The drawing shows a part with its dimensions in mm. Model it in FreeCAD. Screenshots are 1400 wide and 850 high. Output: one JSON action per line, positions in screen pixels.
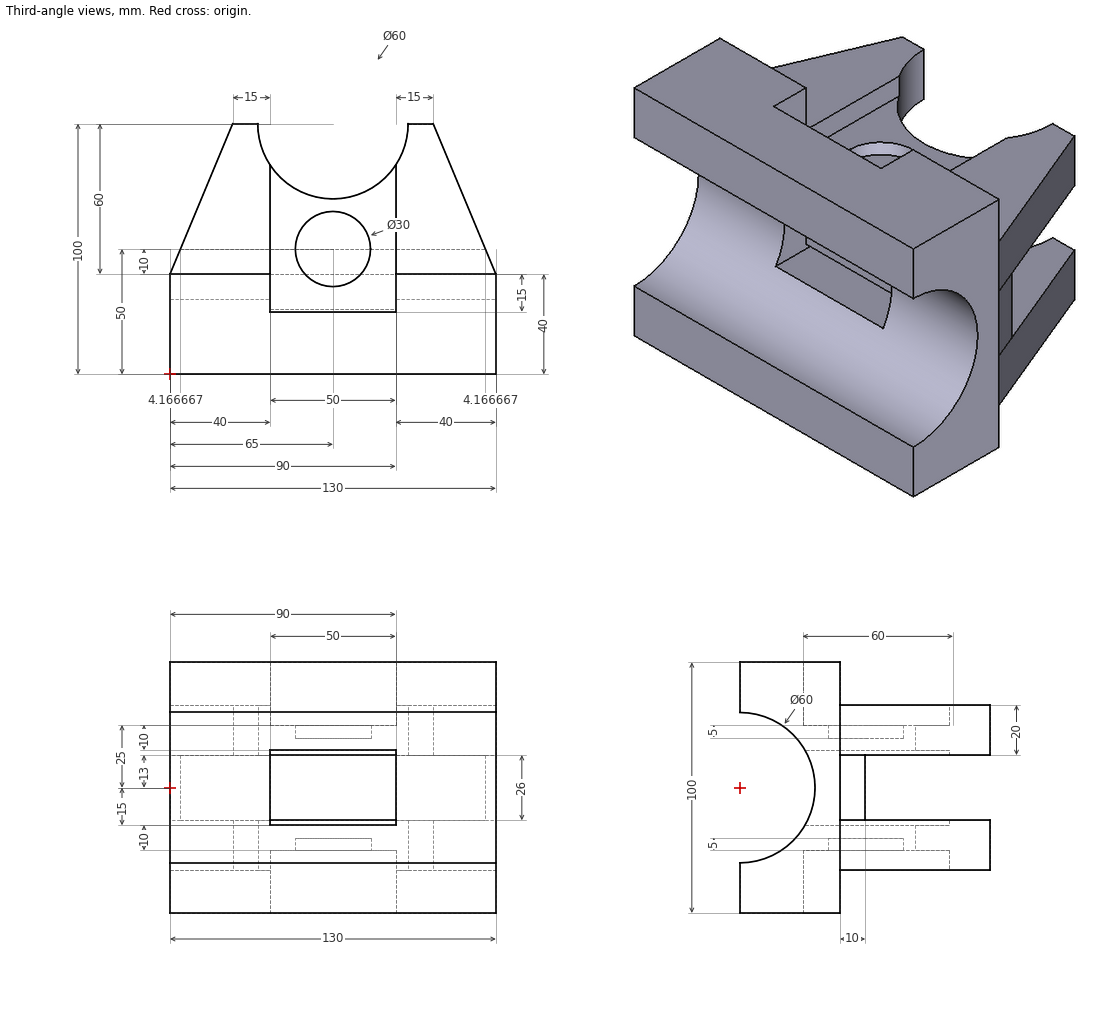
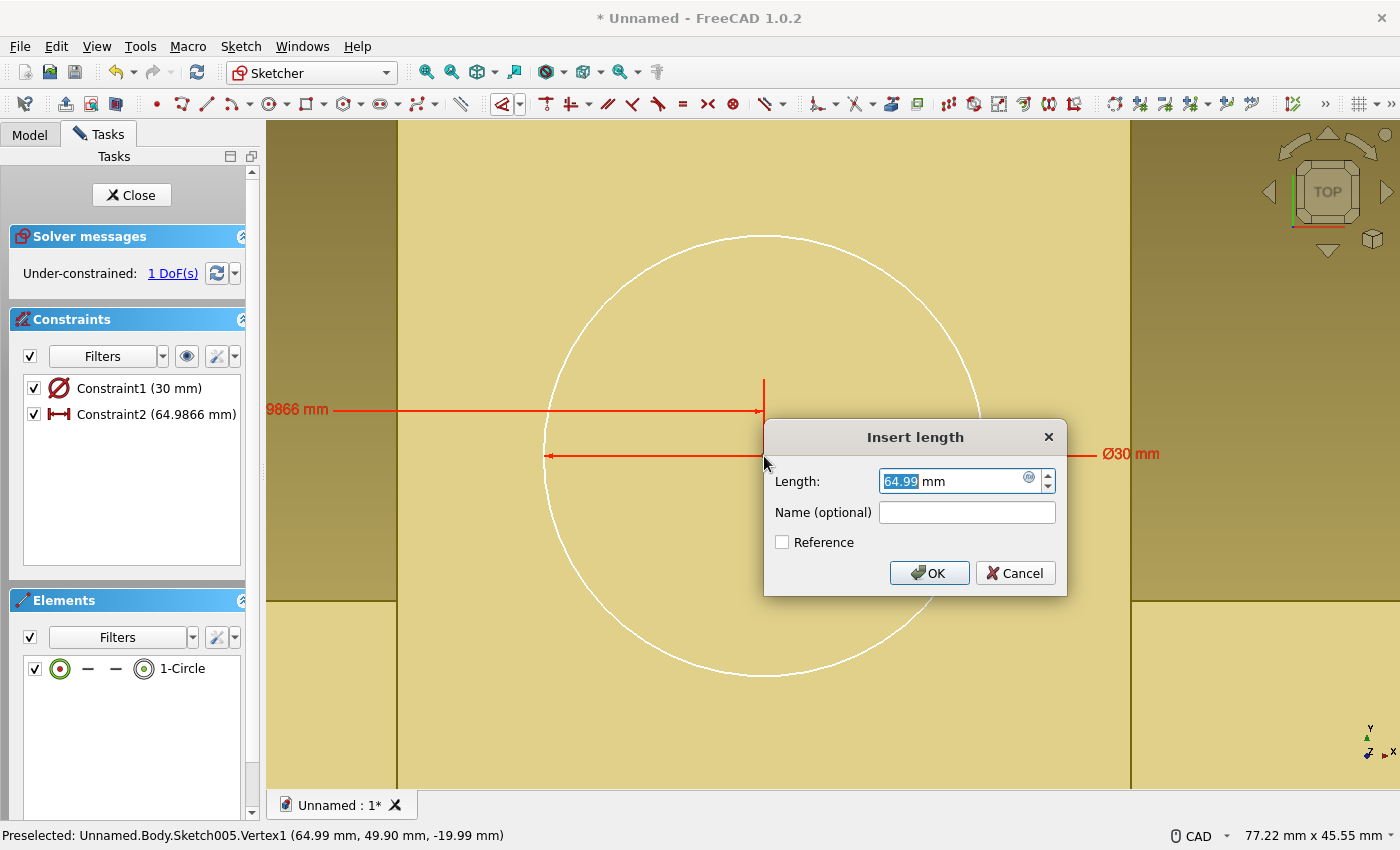
{"action": "type", "text": "65"}
{"action": "key", "text": "Return"}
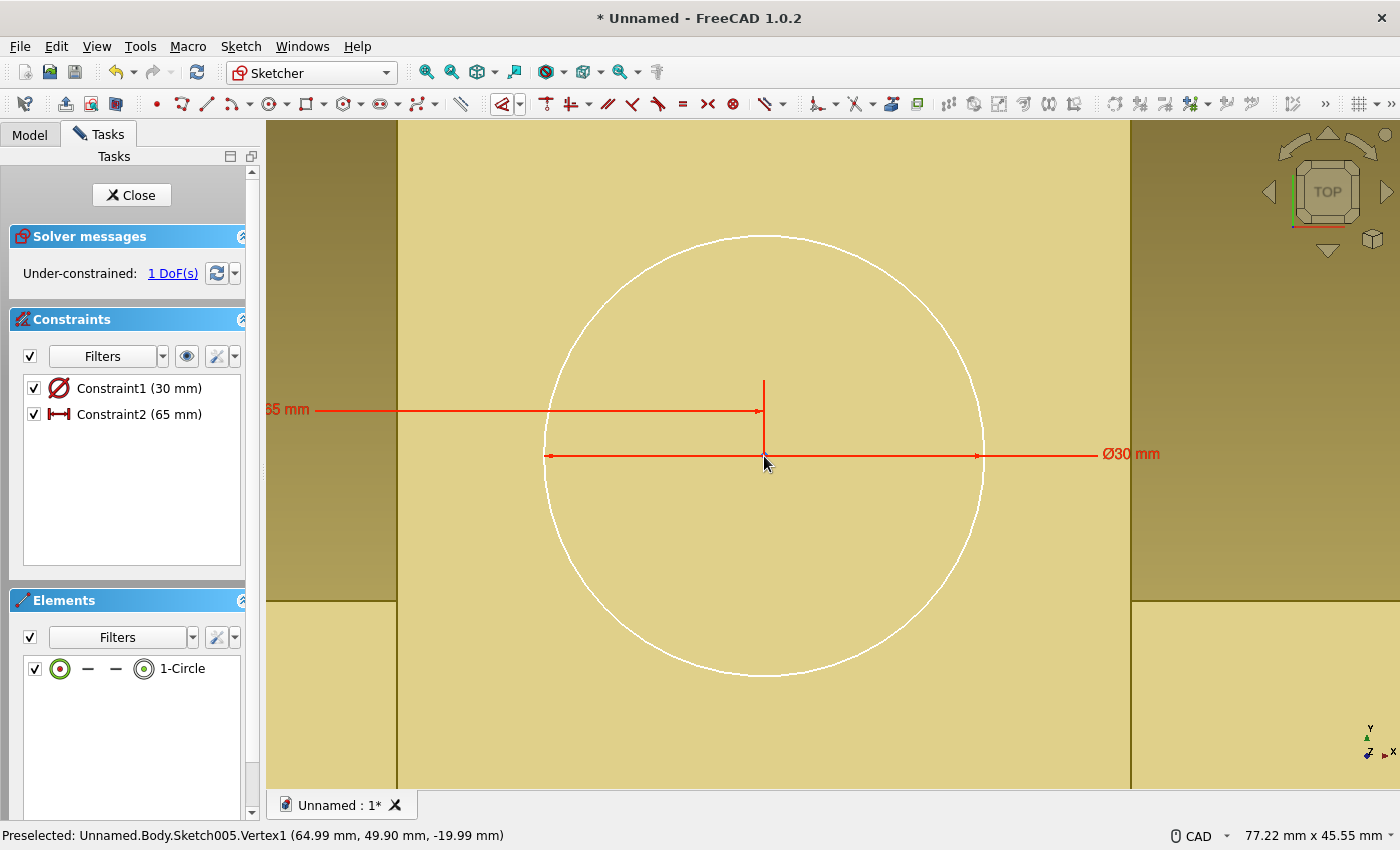
{"action": "left_click", "coordinate": [764, 456]}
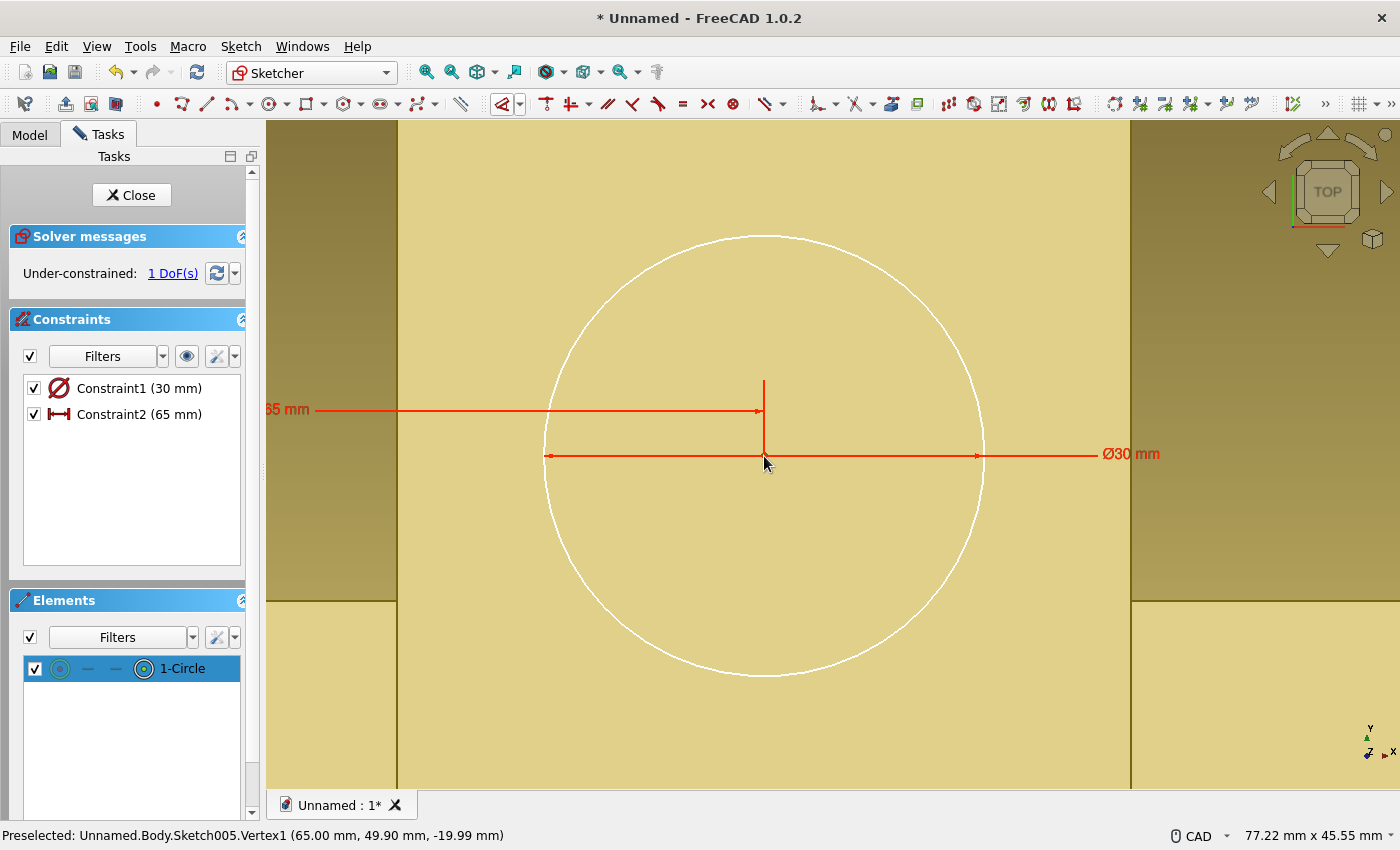
{"action": "key", "text": "i"}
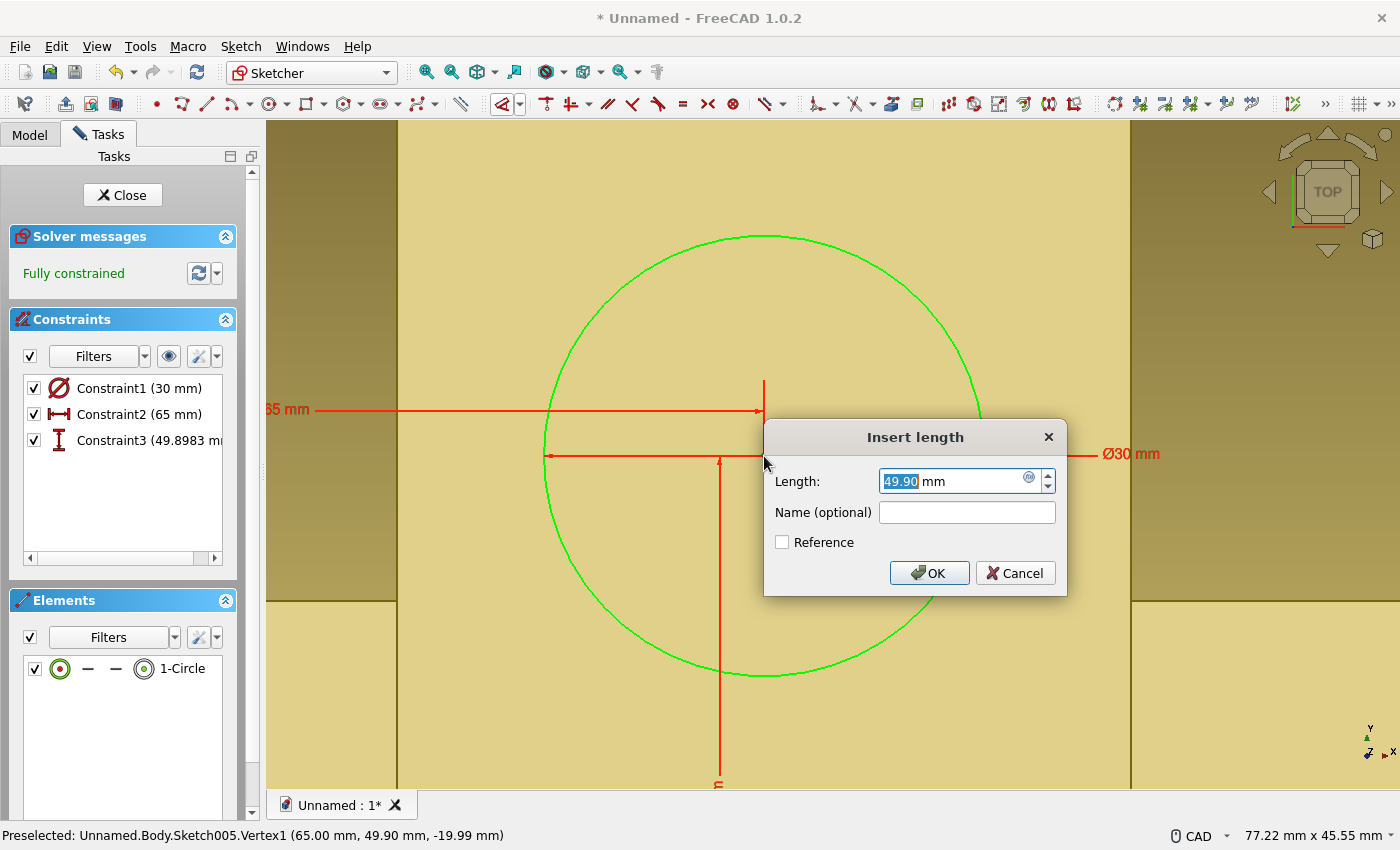
{"action": "type", "text": "50"}
{"action": "key", "text": "Return"}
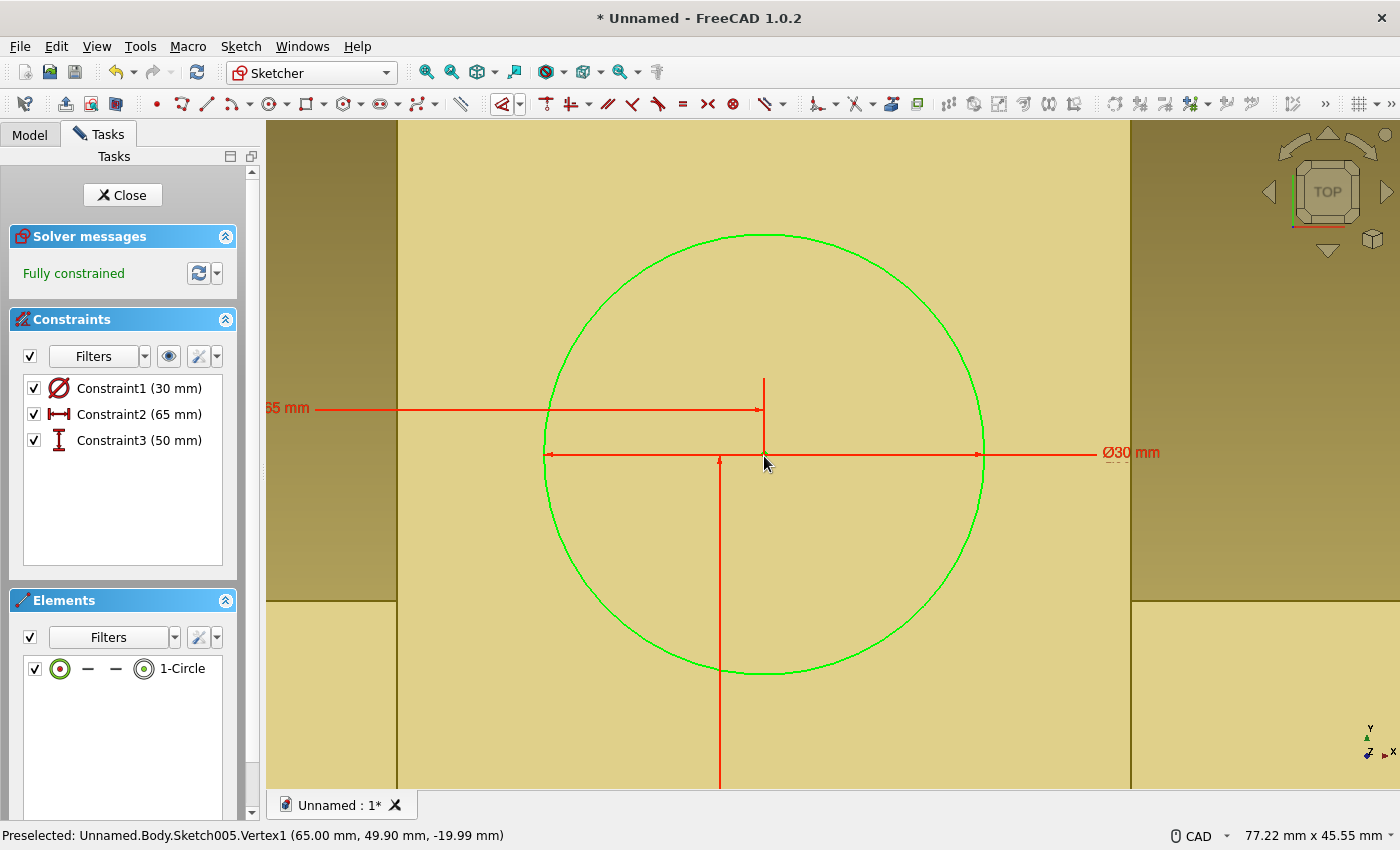
{"action": "left_click", "coordinate": [123, 195]}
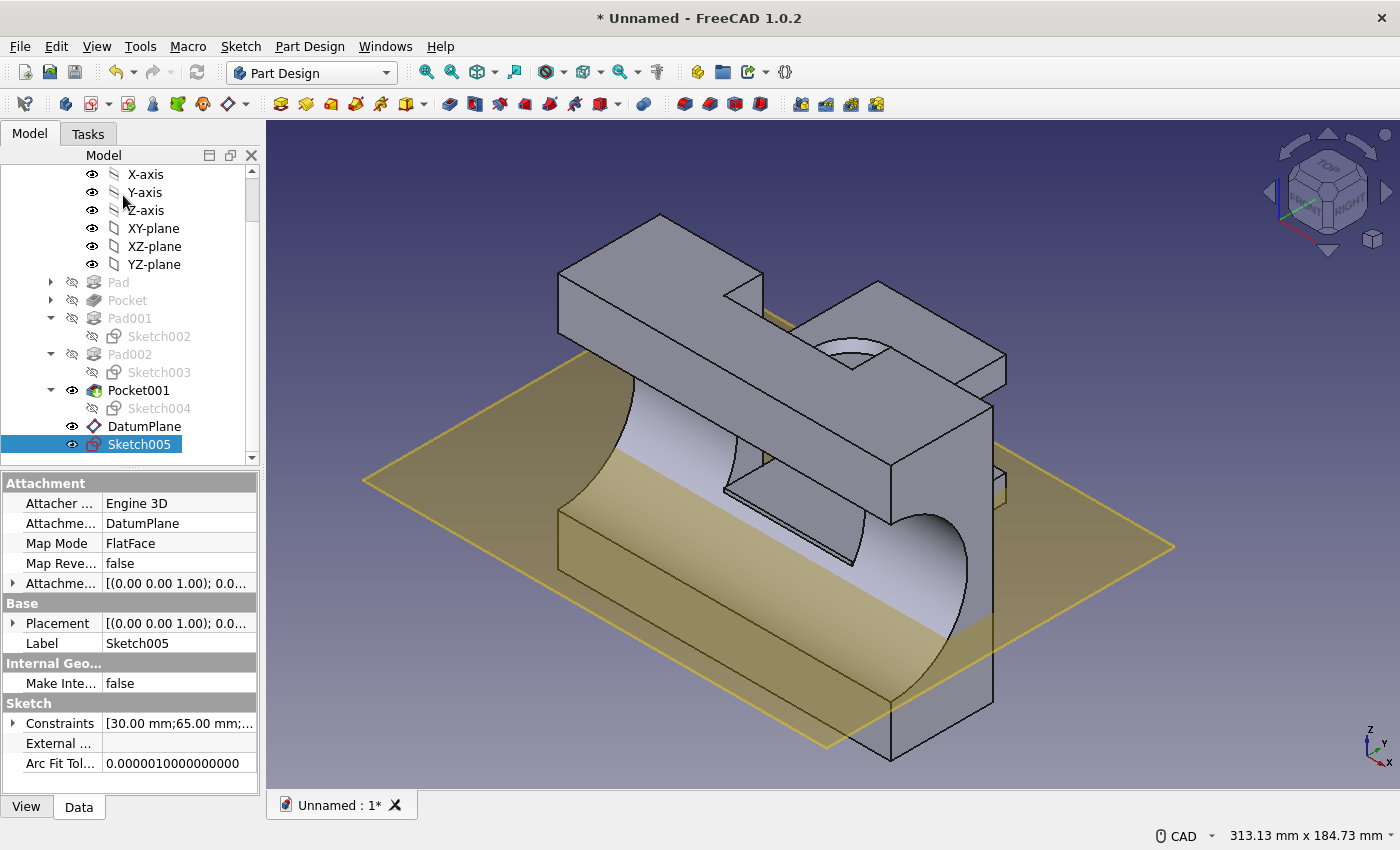
{"action": "left_click", "coordinate": [450, 104]}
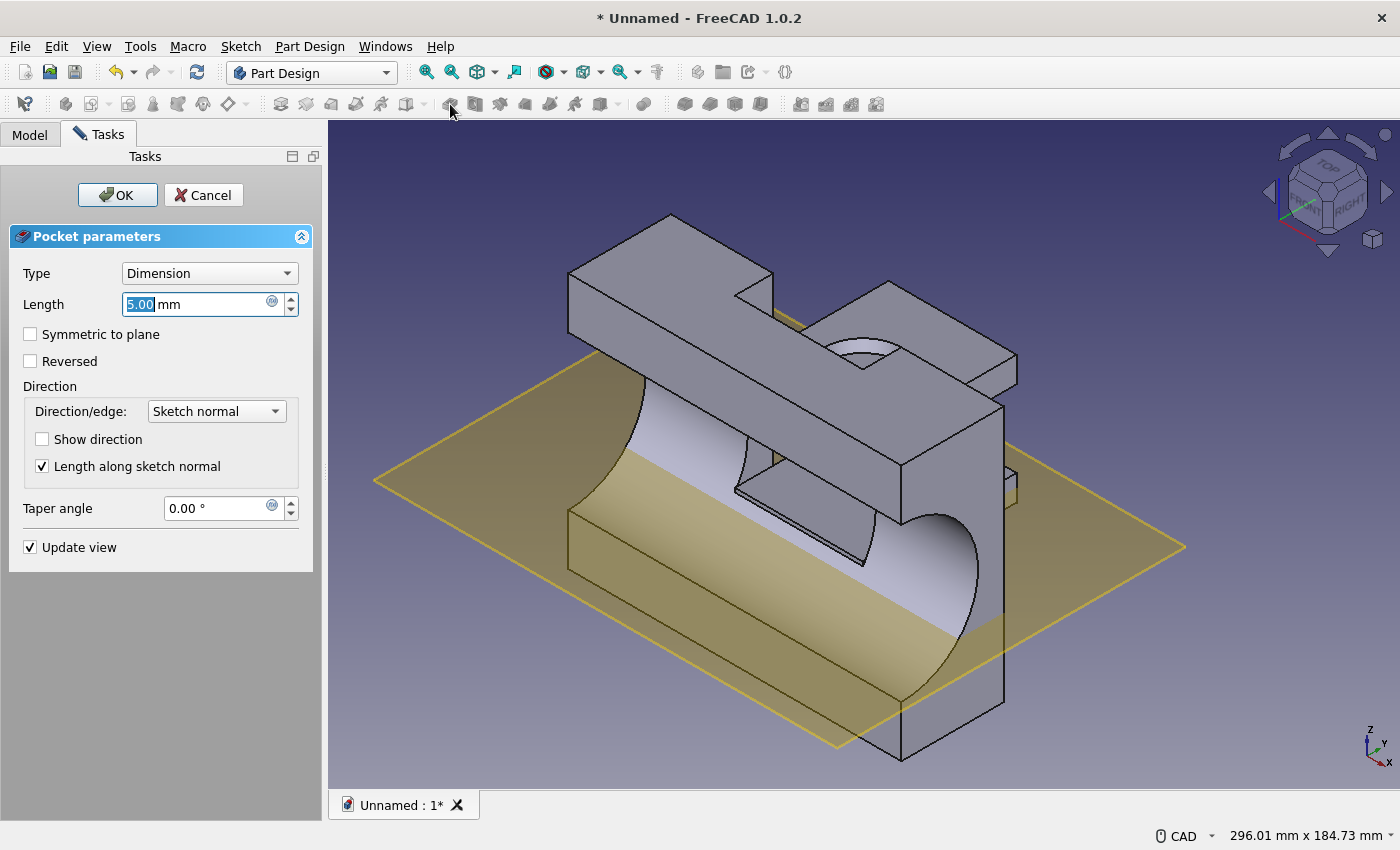
{"action": "type", "text": "5"}
{"action": "key", "text": "Tab"}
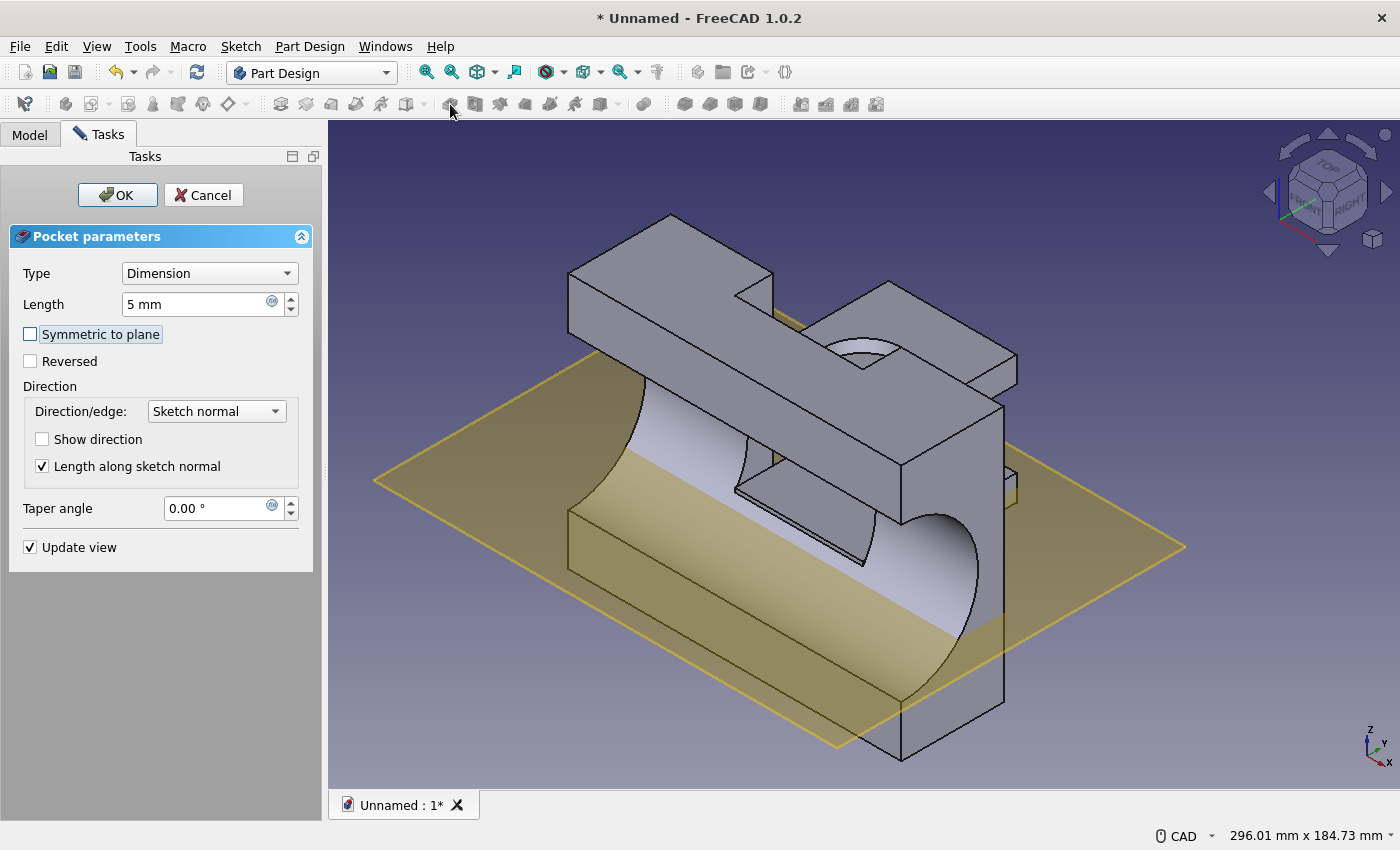
{"action": "left_click", "coordinate": [118, 195]}